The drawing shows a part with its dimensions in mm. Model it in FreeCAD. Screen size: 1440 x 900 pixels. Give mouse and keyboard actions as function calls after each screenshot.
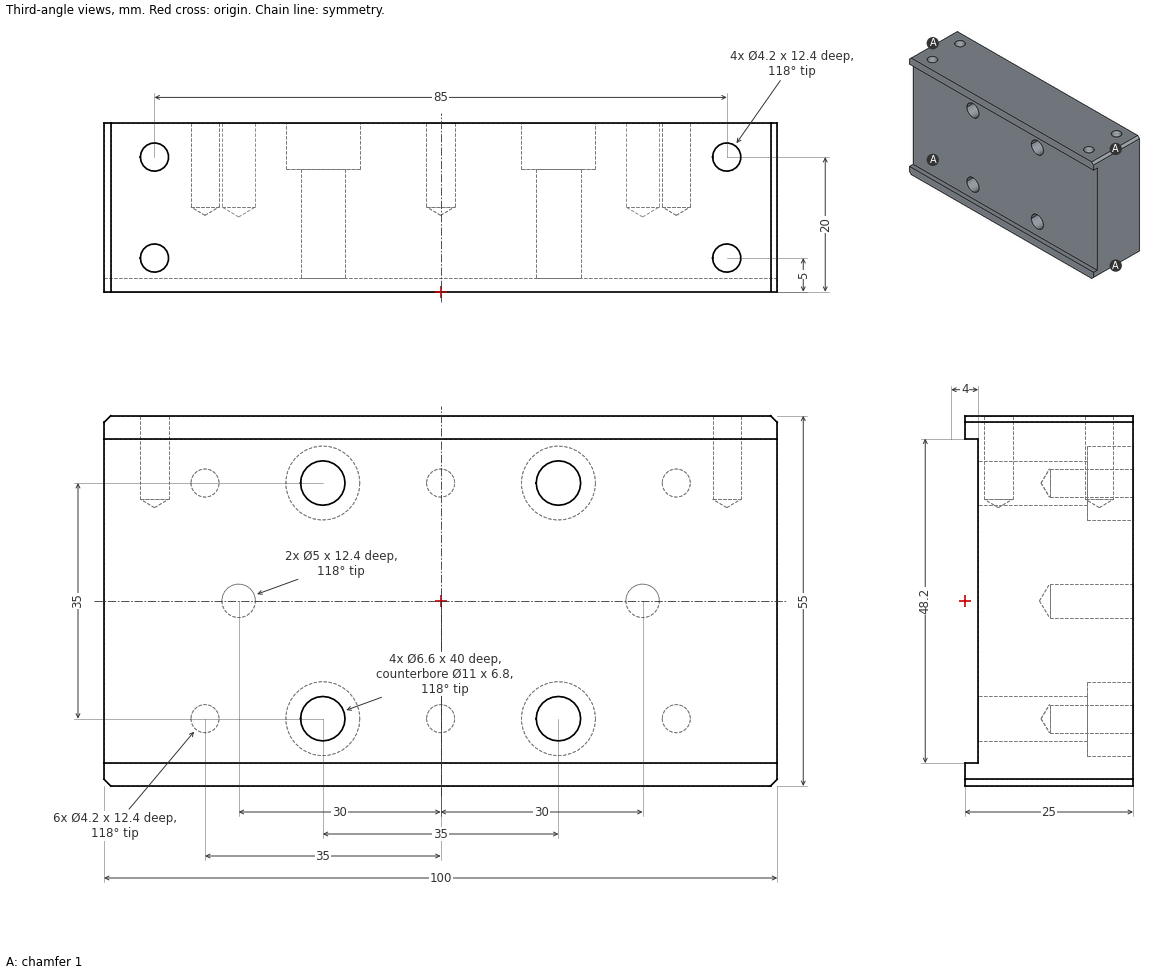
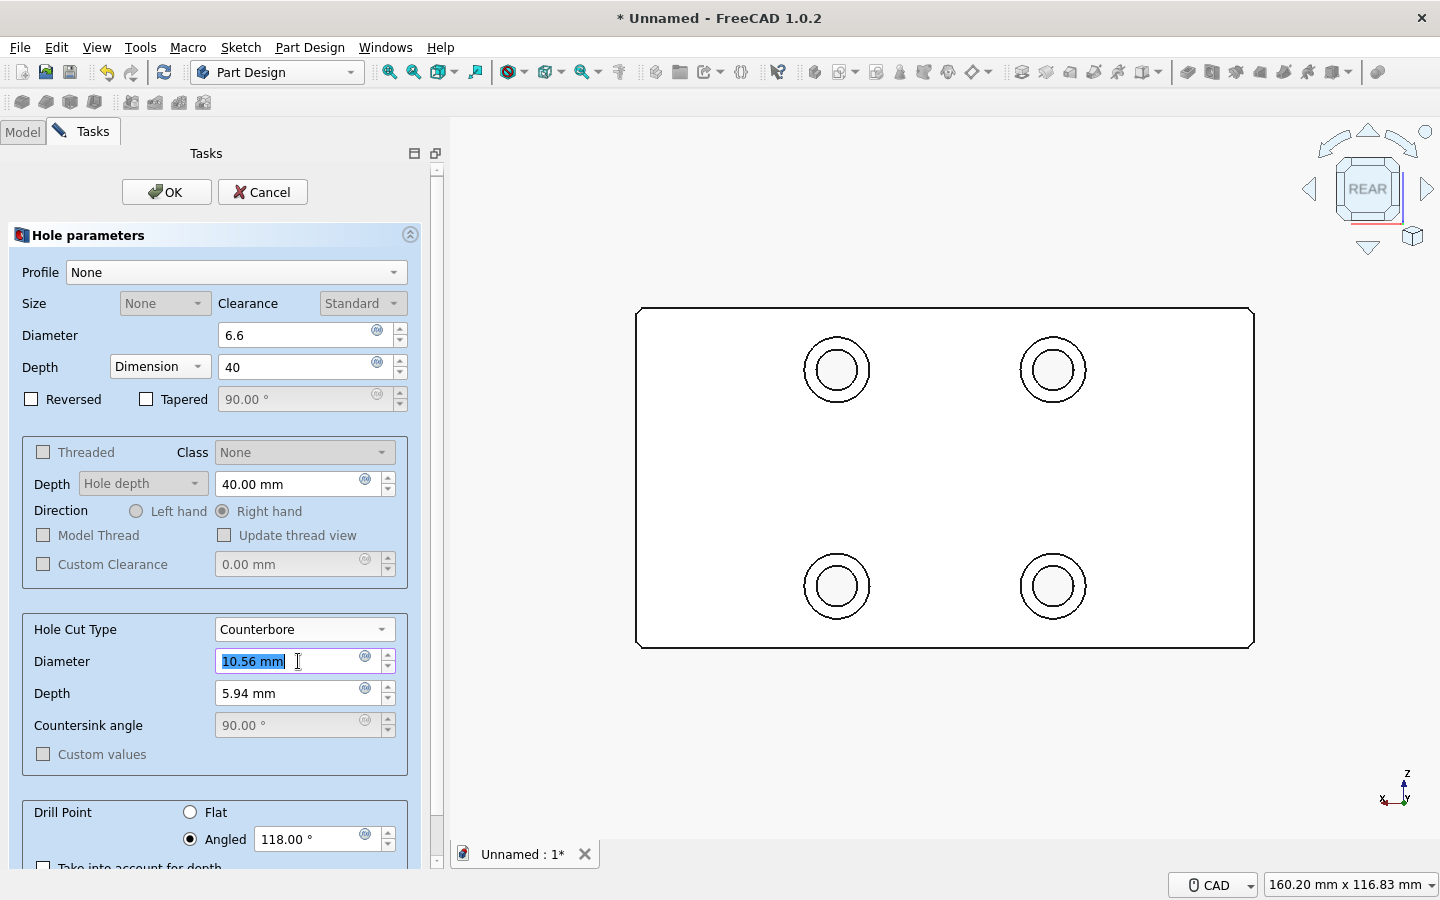
text(11)
key(Tab)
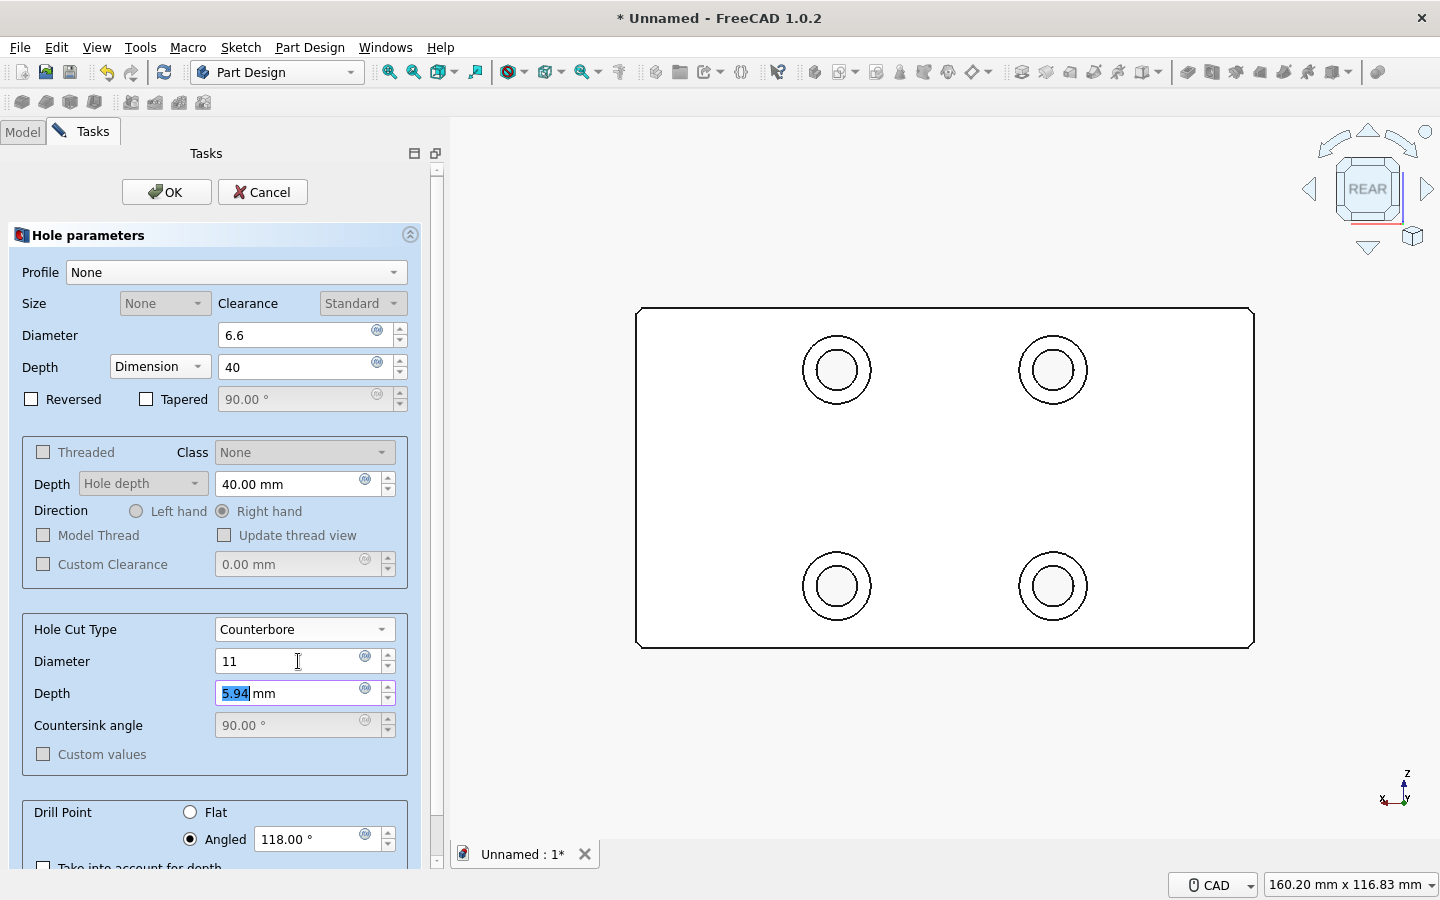
text(6.8)
key(Tab)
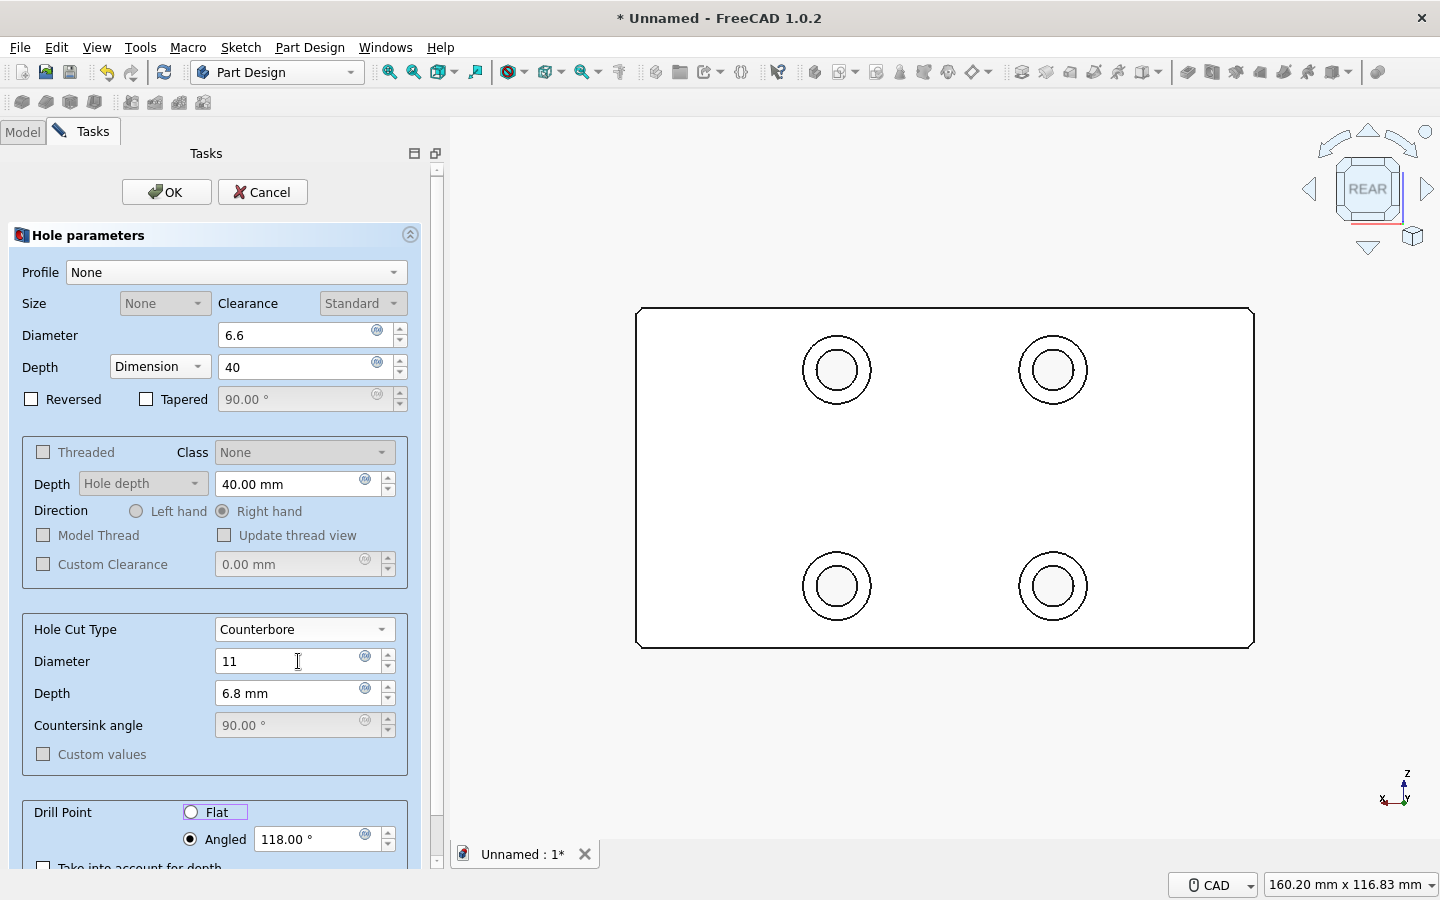
click(167, 192)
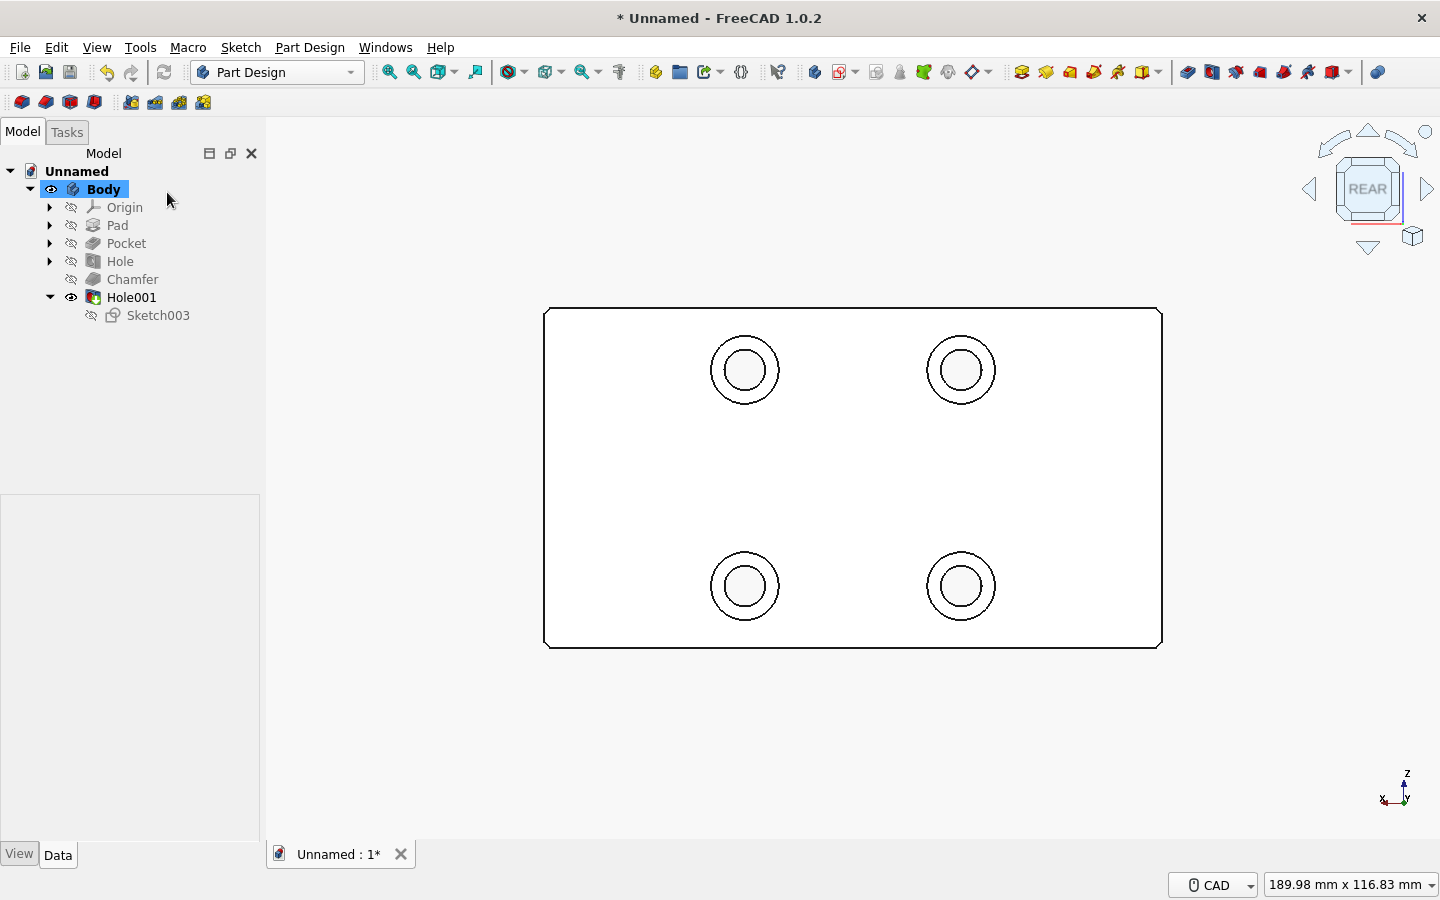
click(853, 477)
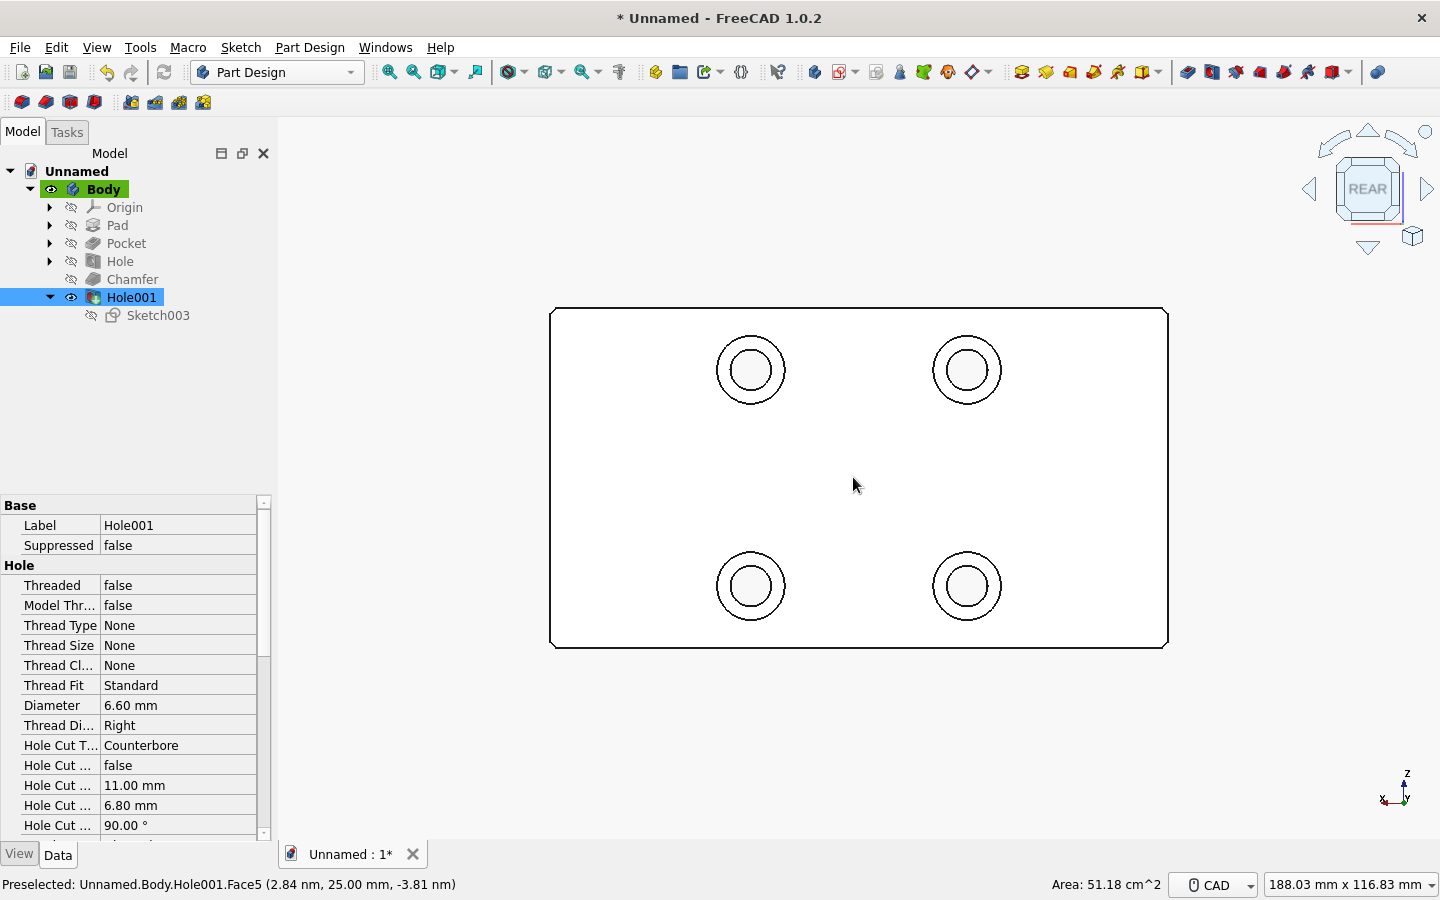
click(840, 72)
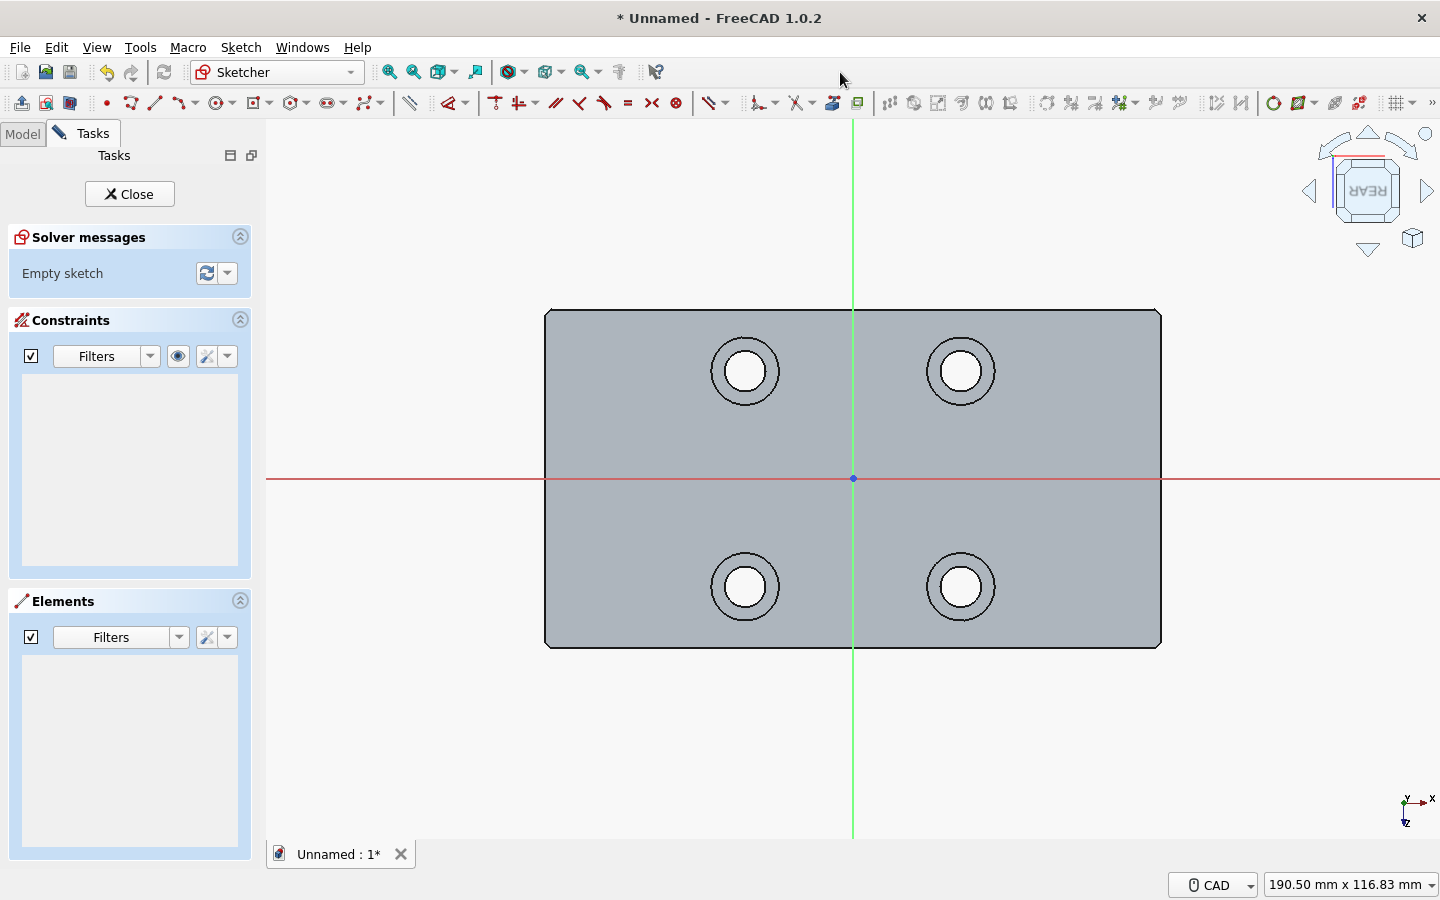
scroll(992, 479, up, 2)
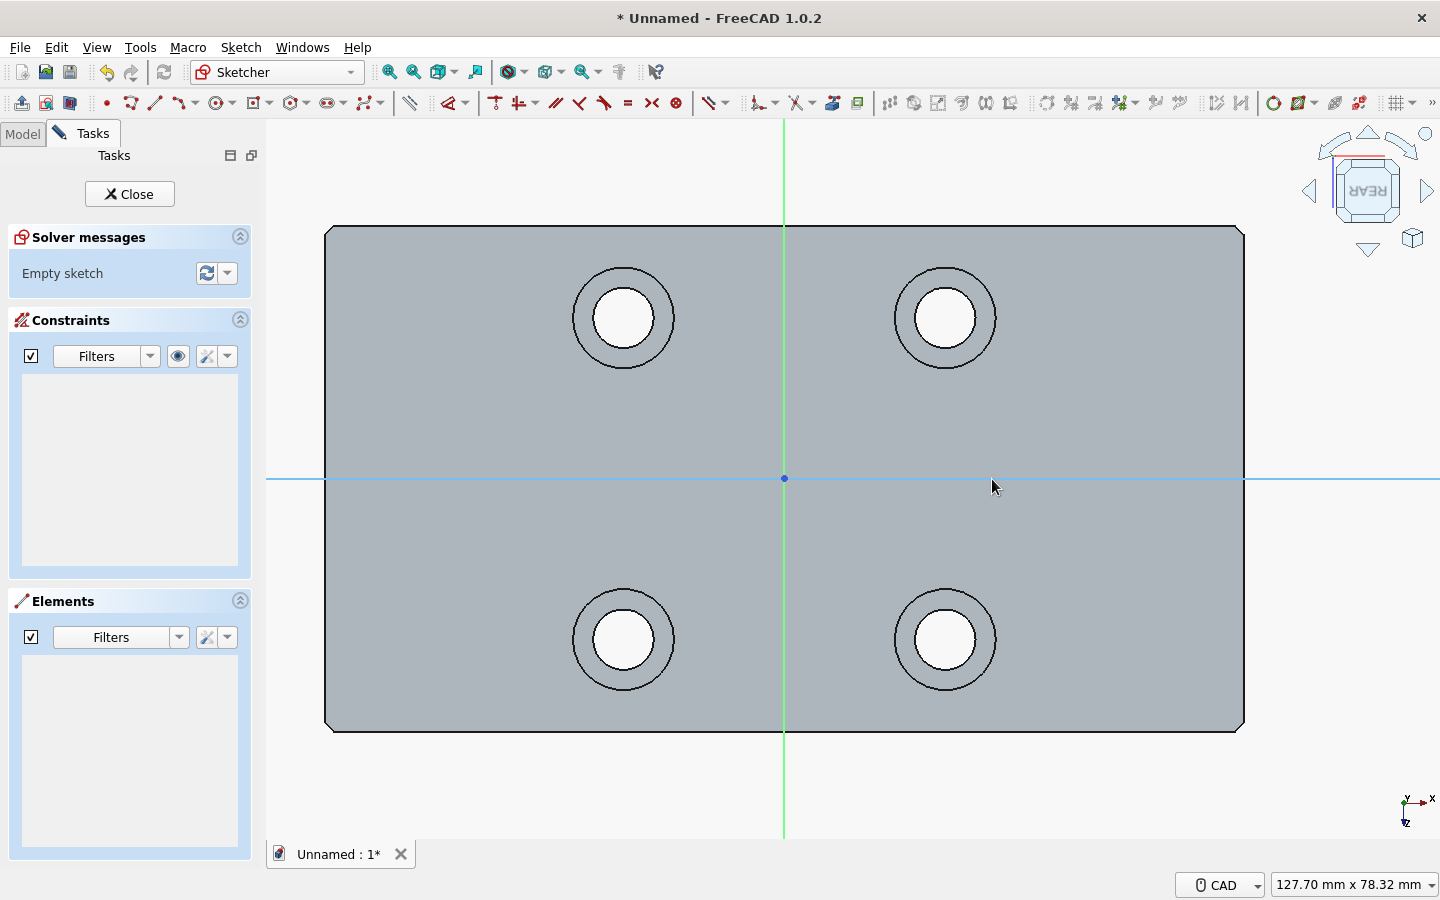
click(216, 104)